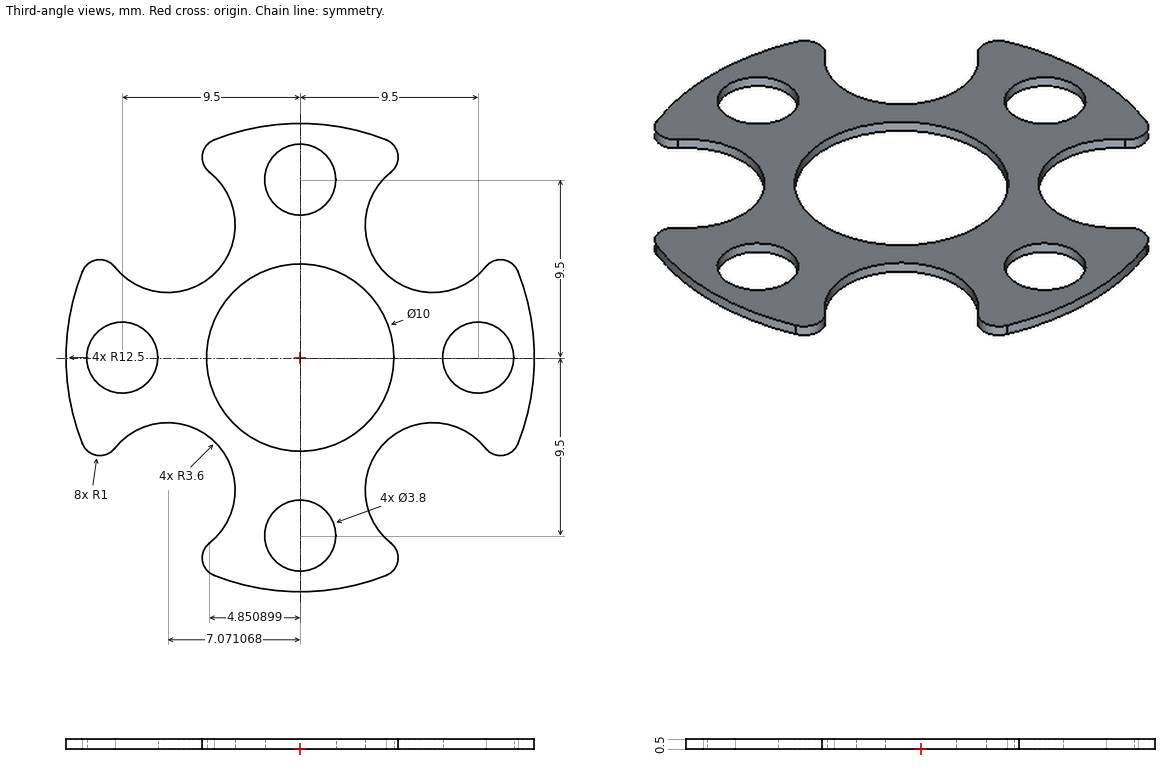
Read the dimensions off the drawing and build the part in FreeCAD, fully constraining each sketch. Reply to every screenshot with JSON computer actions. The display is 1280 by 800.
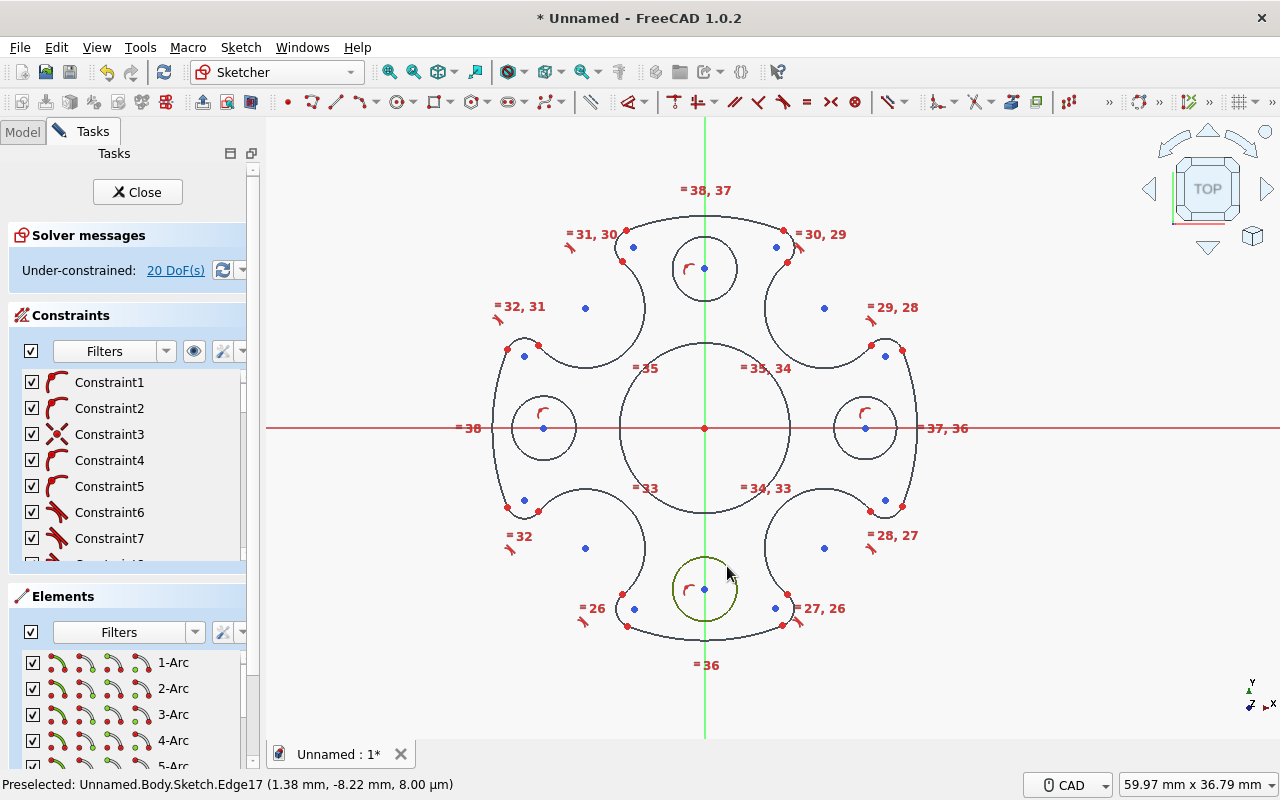
{"action": "left_click", "coordinate": [566, 406]}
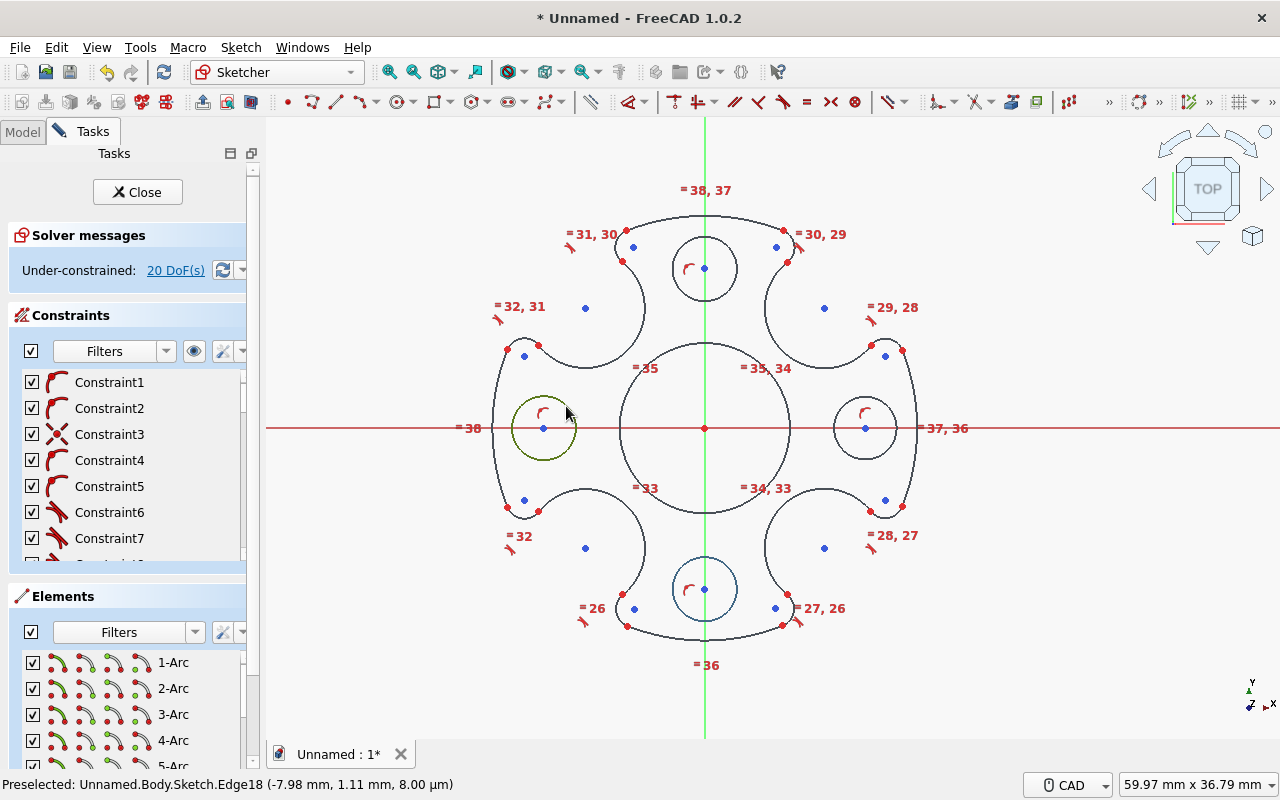
{"action": "left_click", "coordinate": [887, 406]}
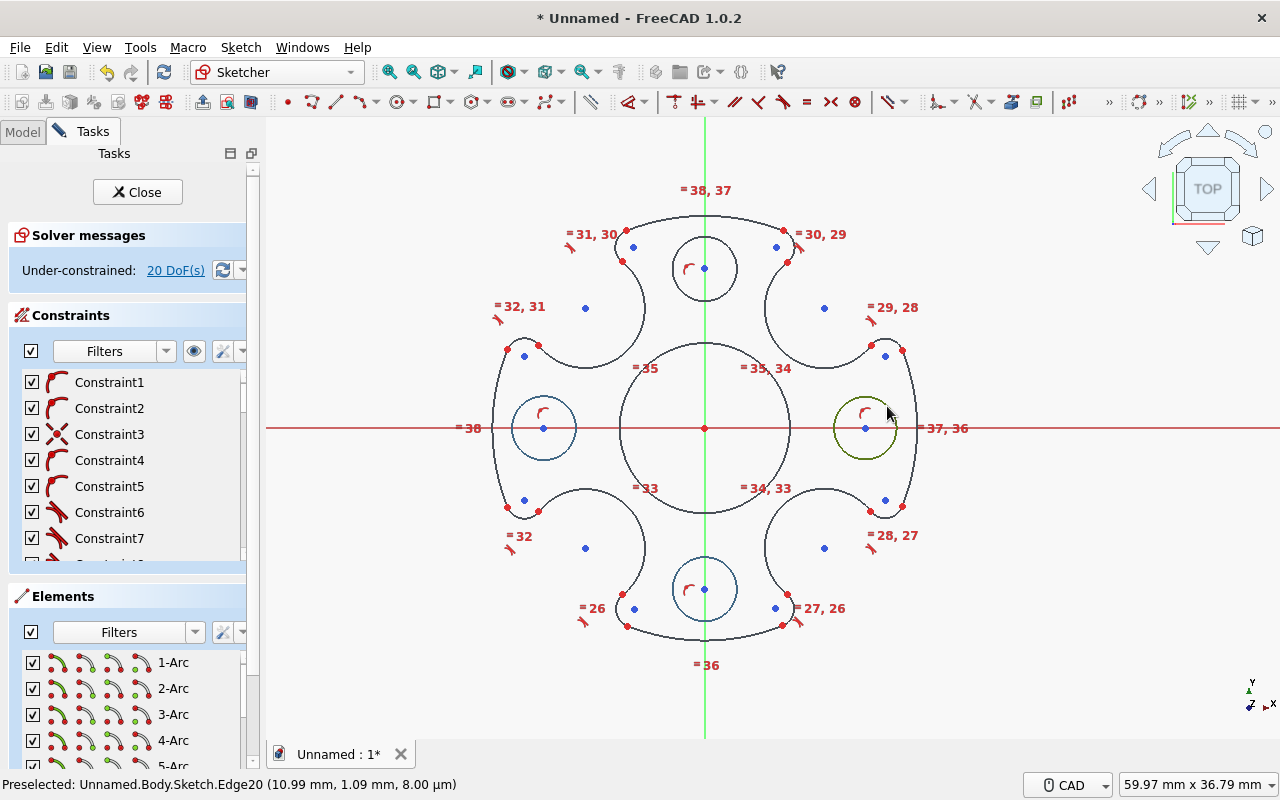
{"action": "left_click", "coordinate": [727, 246]}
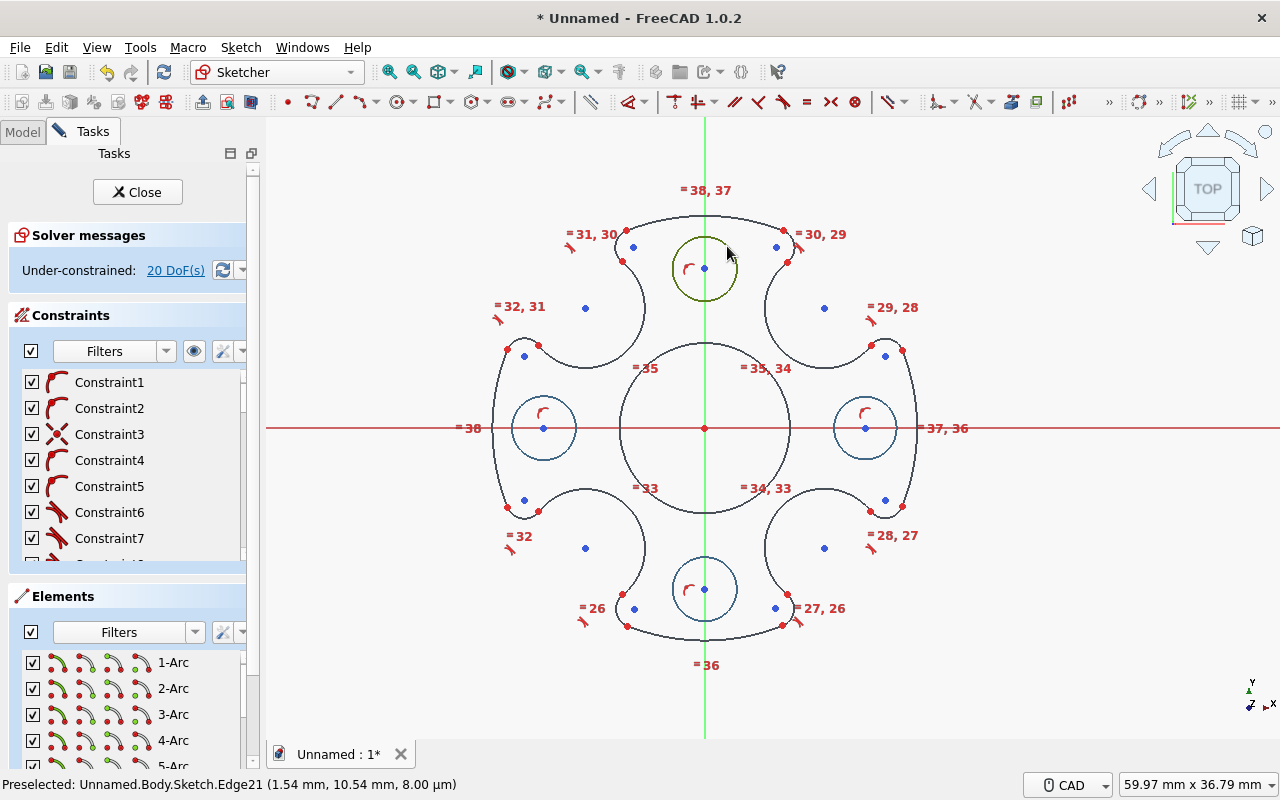
{"action": "key", "text": "e"}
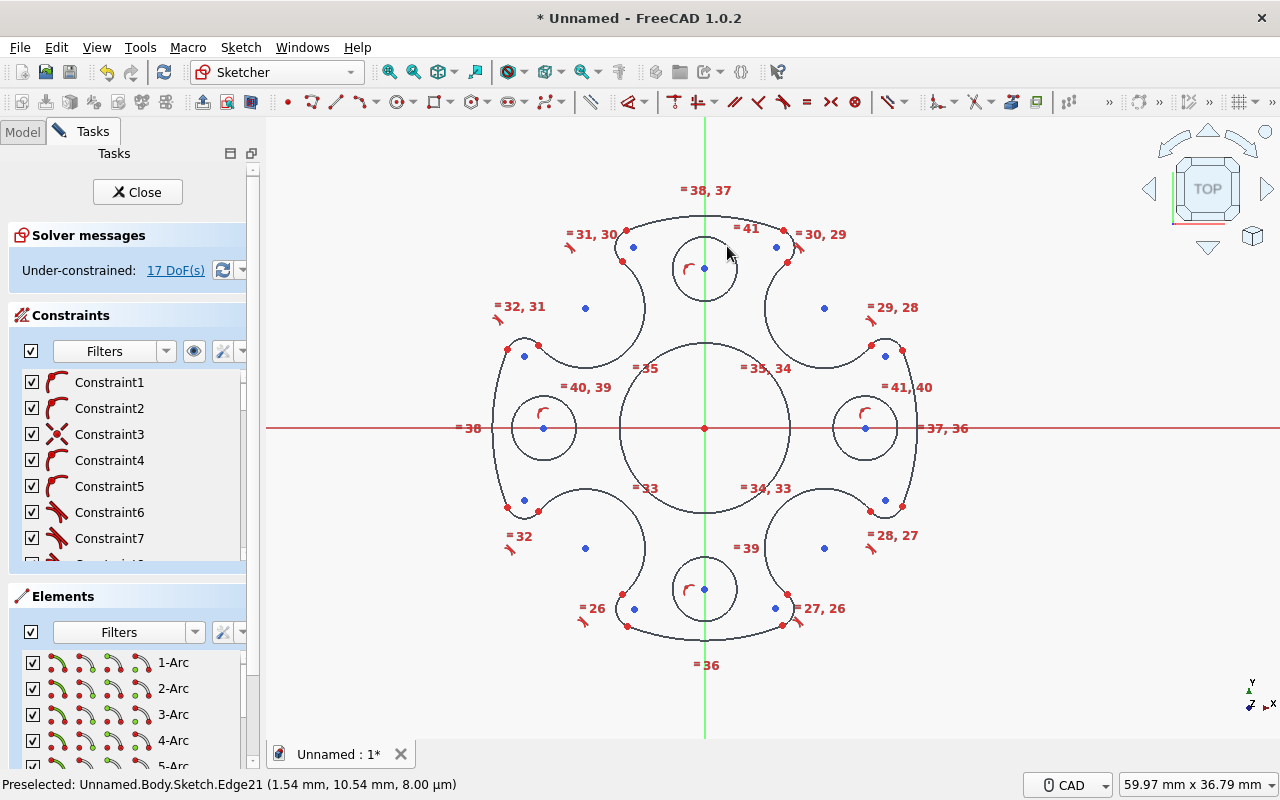
{"action": "left_click", "coordinate": [586, 549]}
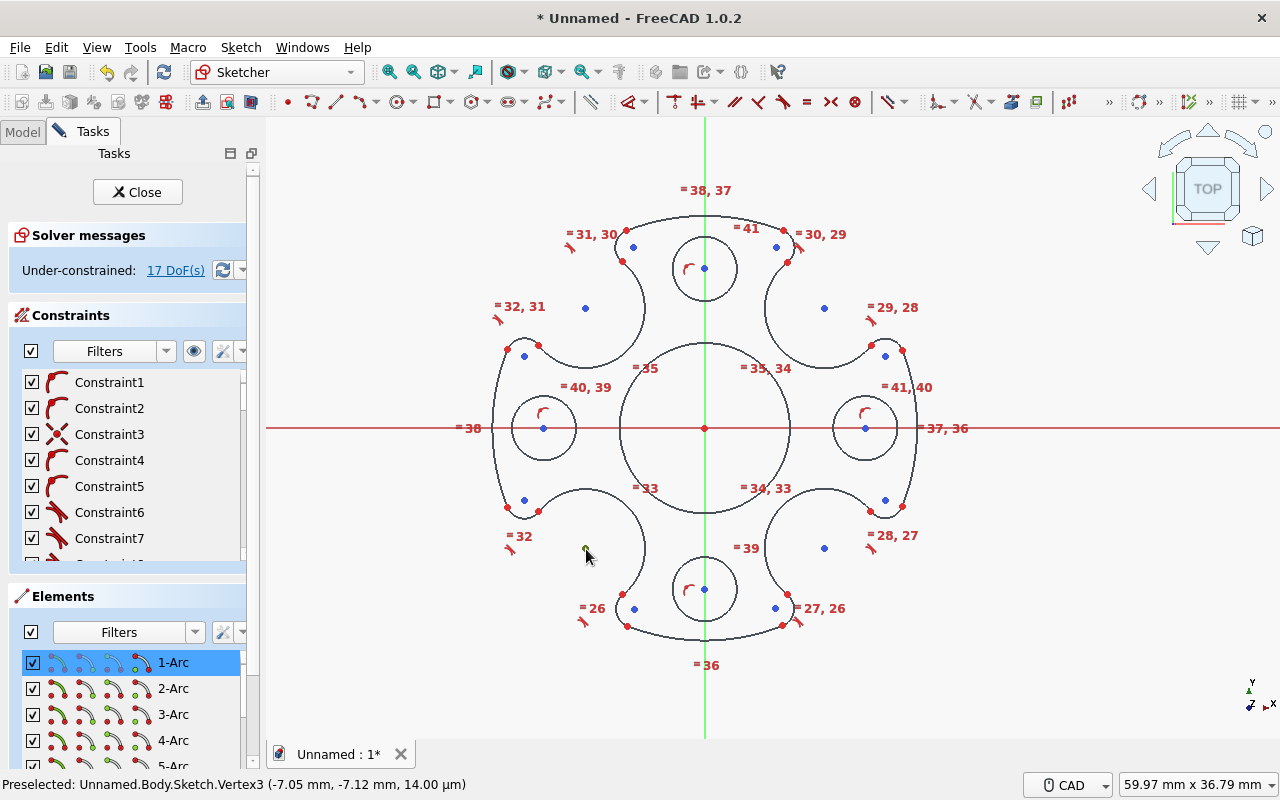
{"action": "left_click", "coordinate": [824, 548]}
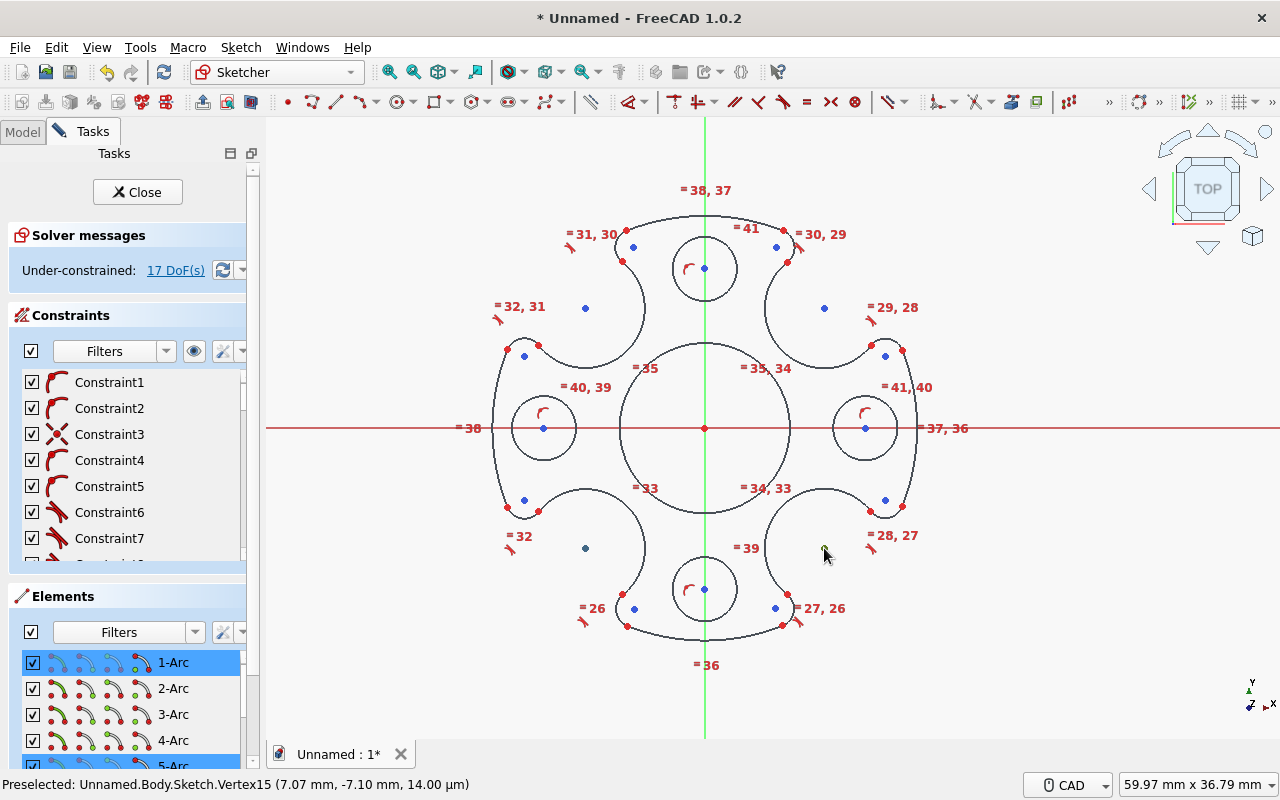
{"action": "left_click", "coordinate": [705, 468]}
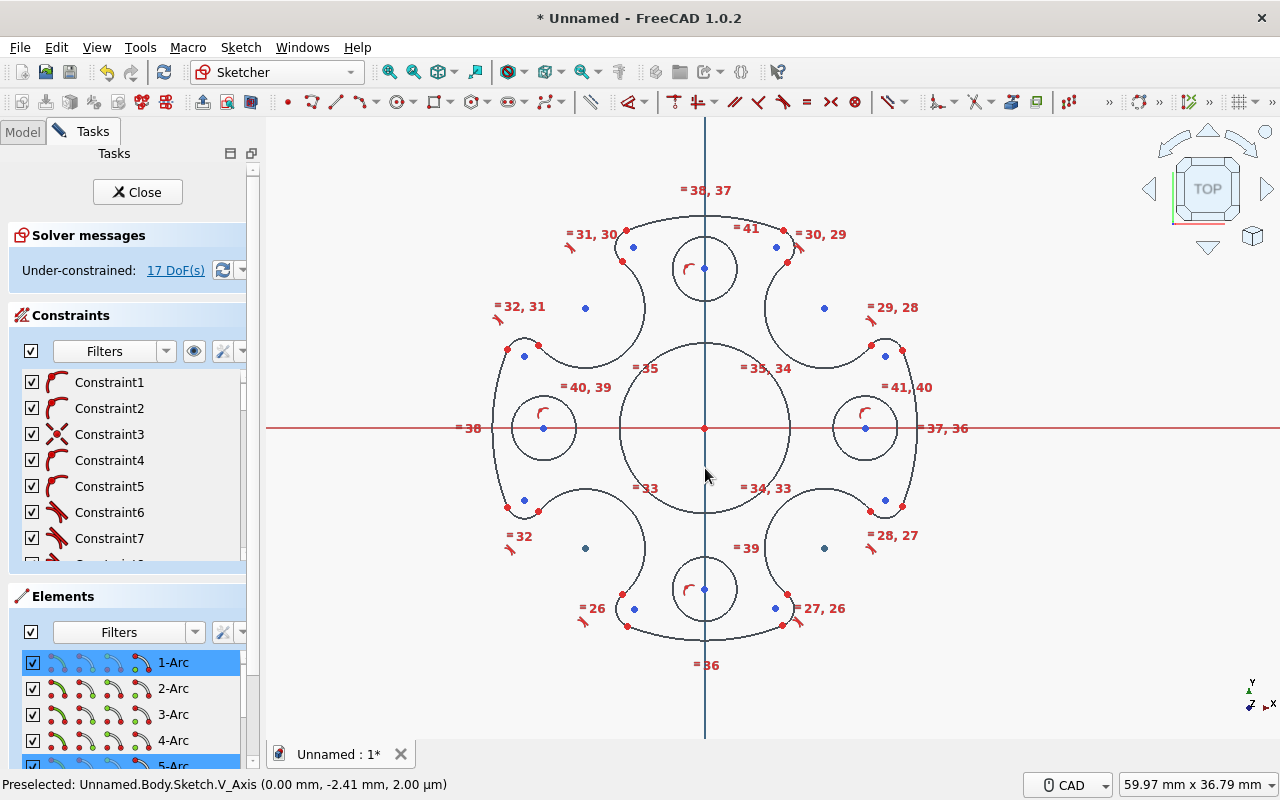
{"action": "left_click", "coordinate": [832, 102]}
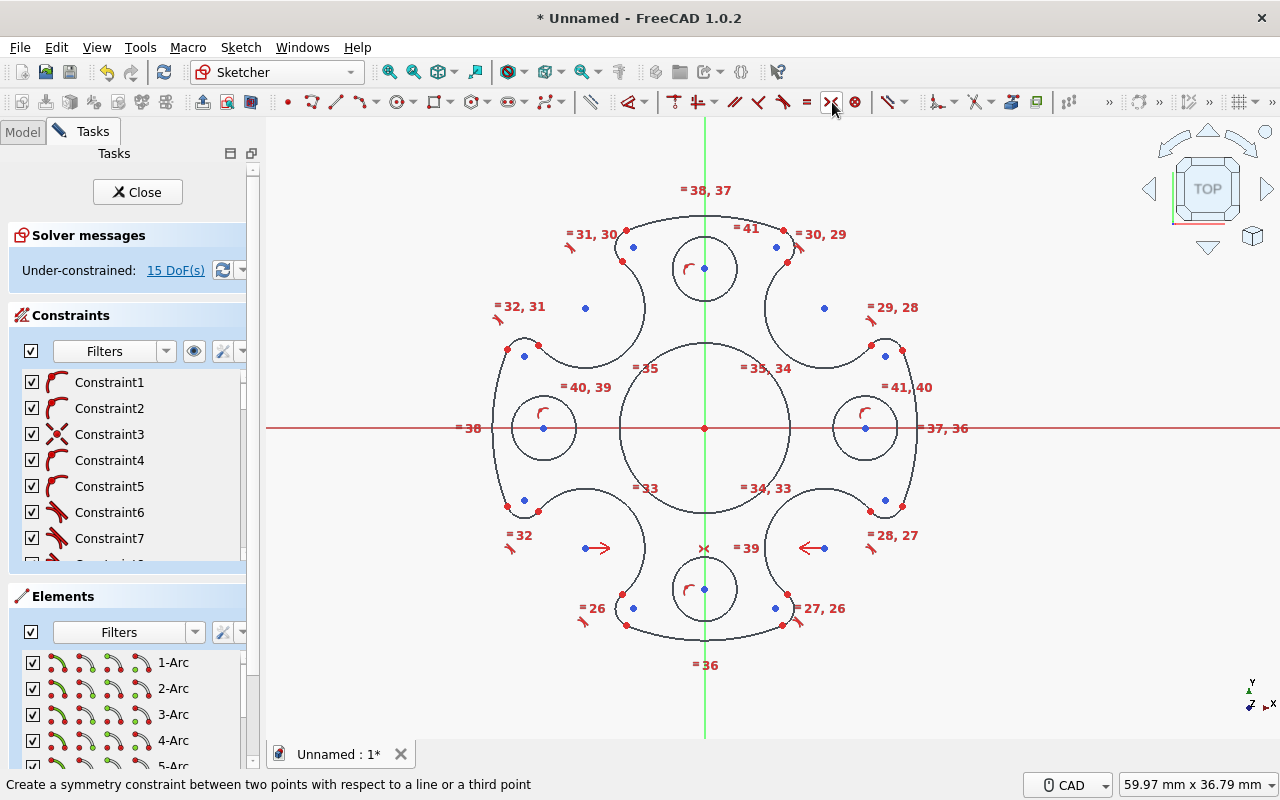
{"action": "left_click", "coordinate": [824, 548]}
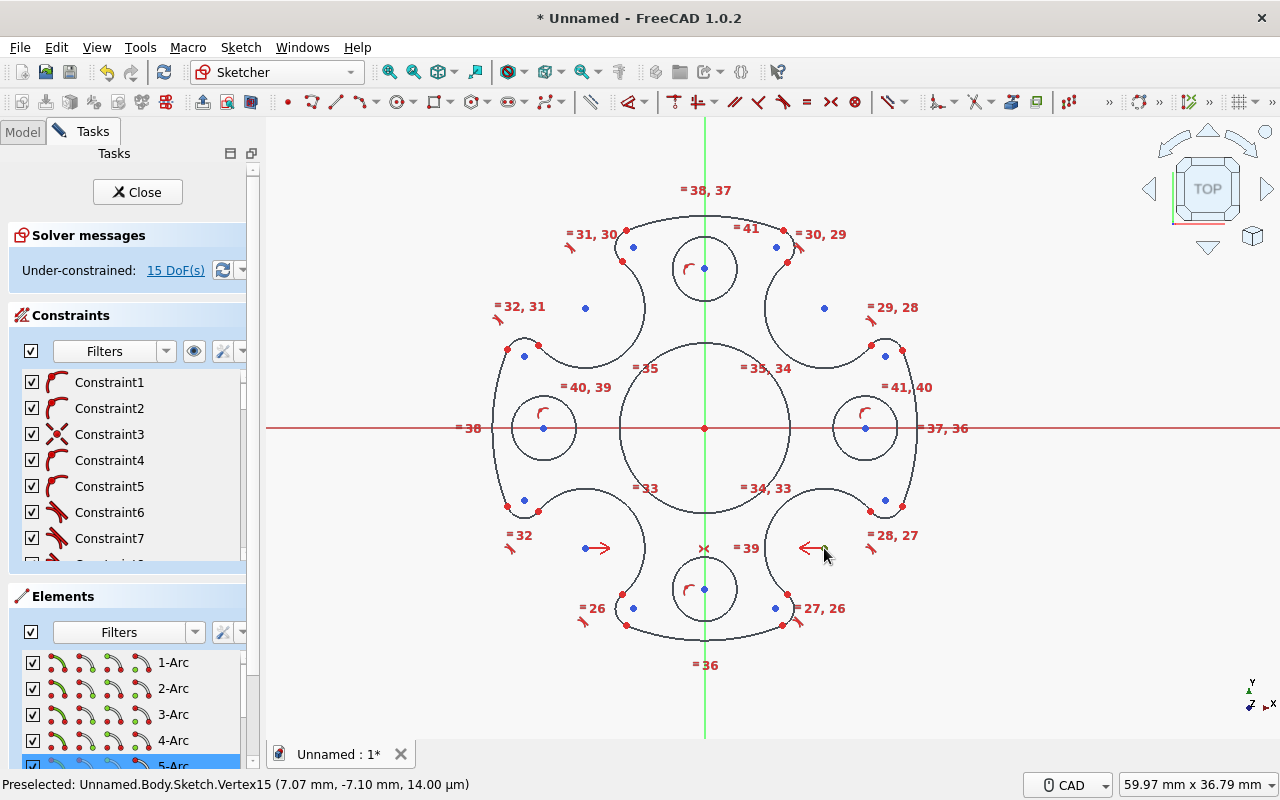
{"action": "left_click", "coordinate": [824, 309]}